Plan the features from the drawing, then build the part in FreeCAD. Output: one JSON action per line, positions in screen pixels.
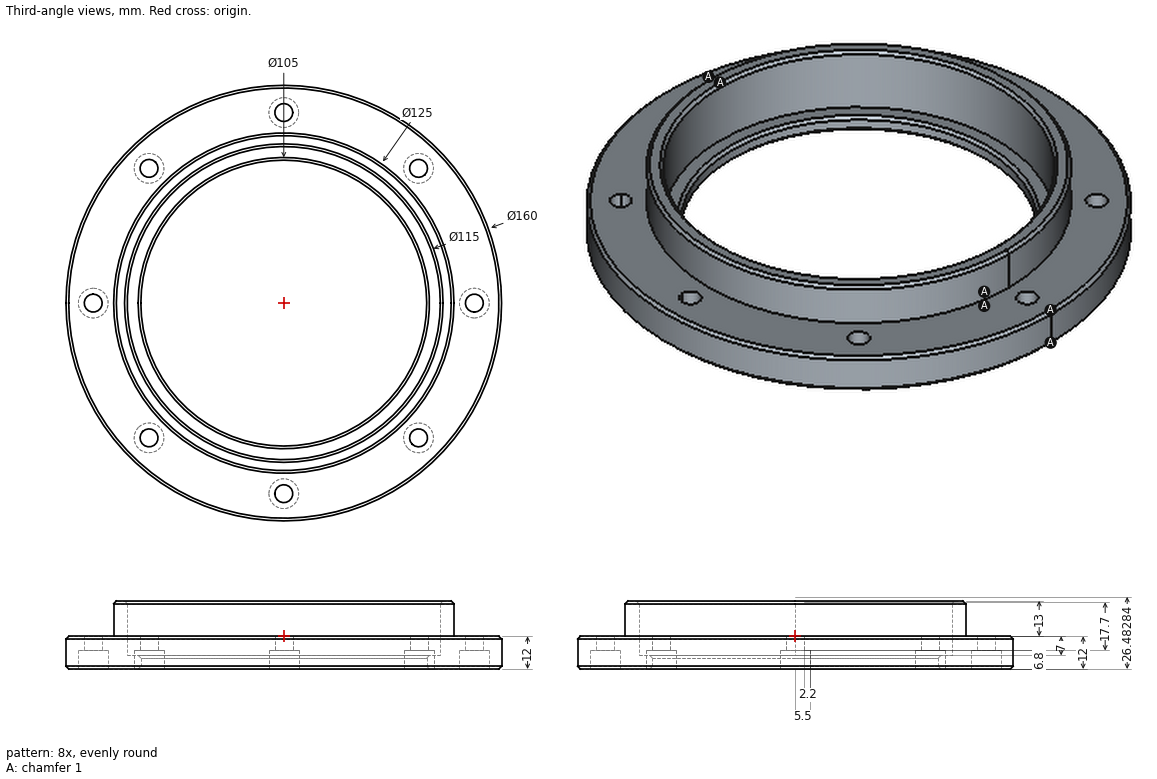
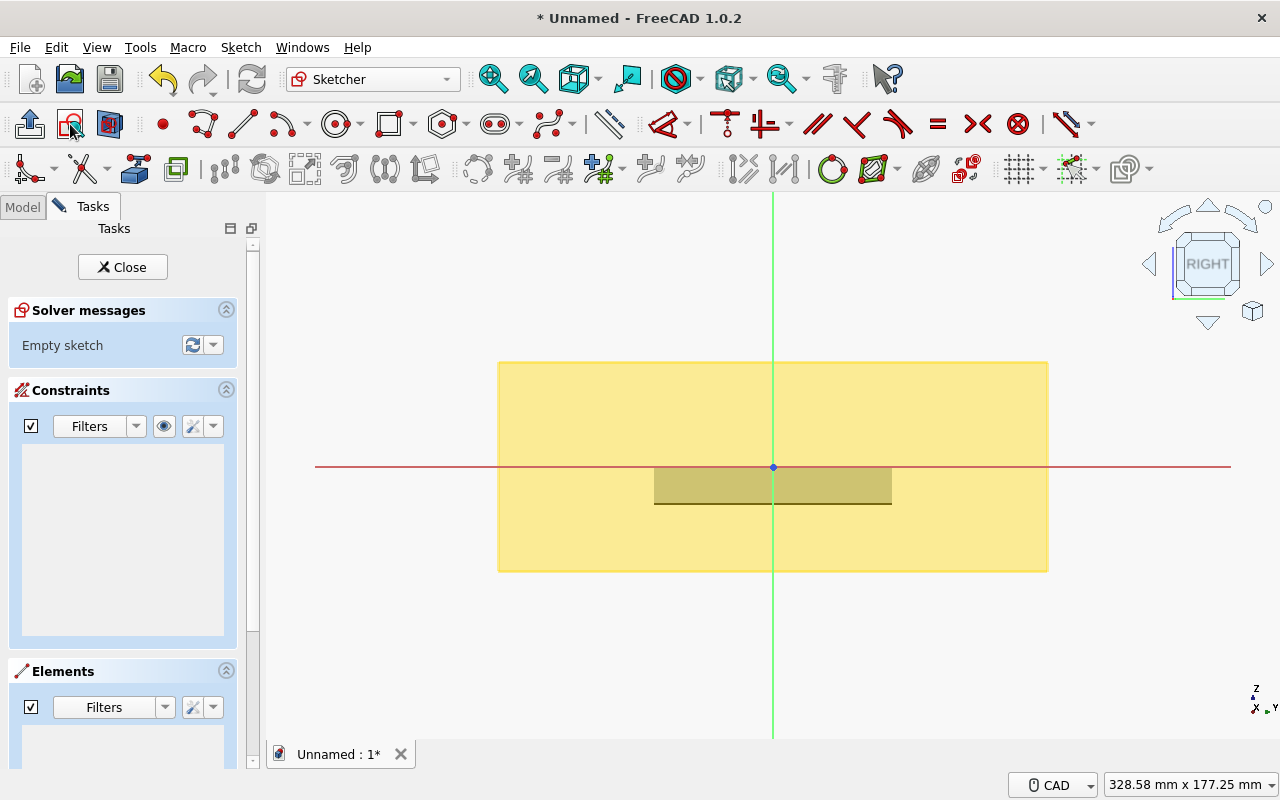
{"action": "scroll", "coordinate": [807, 462], "scroll_direction": "up", "scroll_amount": 7}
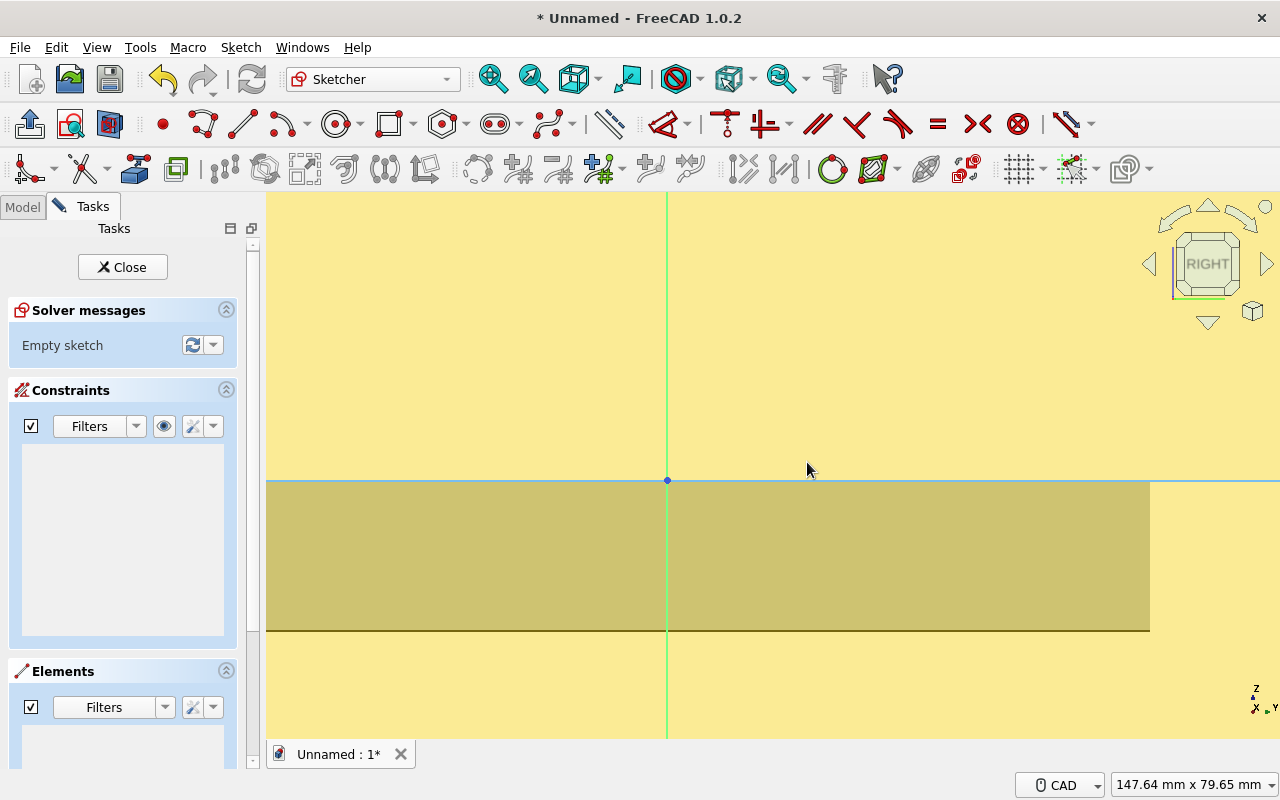
{"action": "key", "text": "g m"}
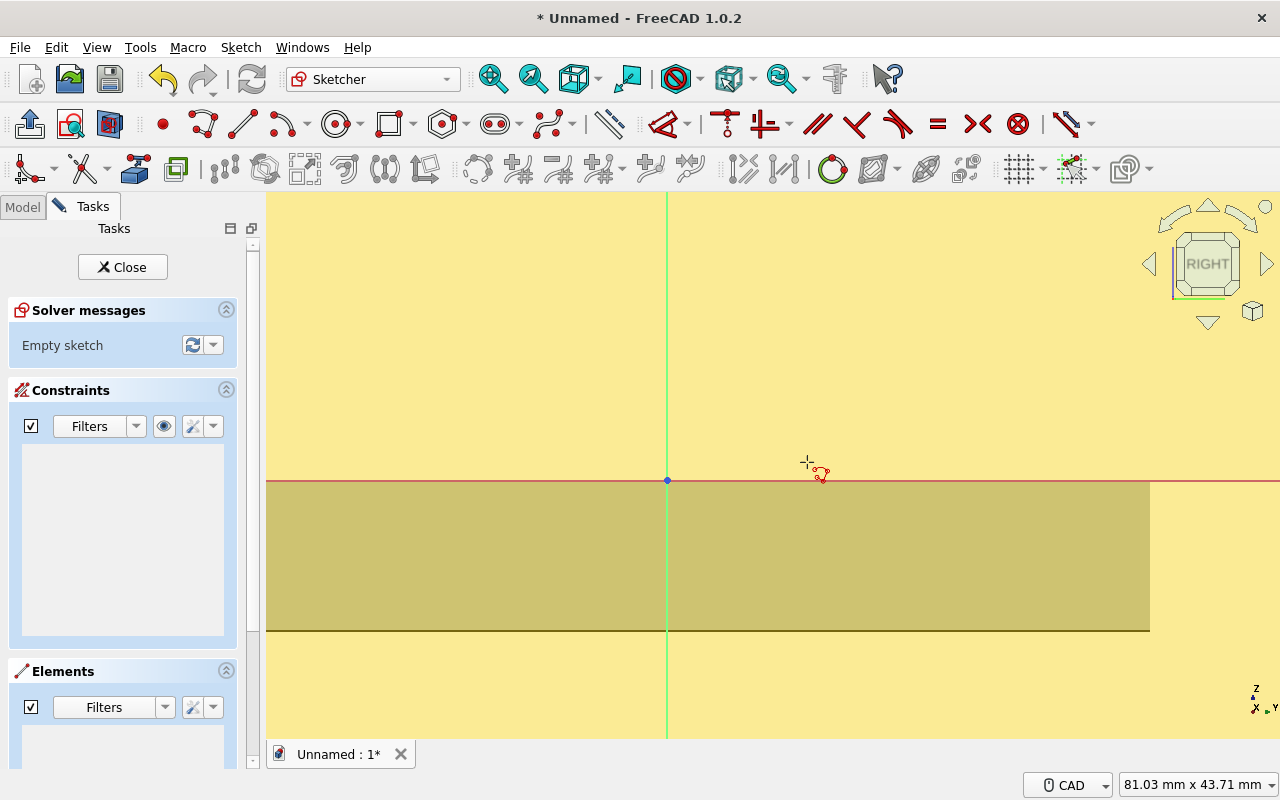
{"action": "left_click", "coordinate": [709, 546]}
{"action": "left_click", "coordinate": [709, 325]}
{"action": "left_click", "coordinate": [667, 300]}
{"action": "left_click", "coordinate": [676, 631]}
{"action": "left_click", "coordinate": [736, 631]}
{"action": "left_click", "coordinate": [736, 546]}
{"action": "left_click", "coordinate": [709, 547]}
{"action": "key", "text": "Escape"}
{"action": "key", "text": "Escape"}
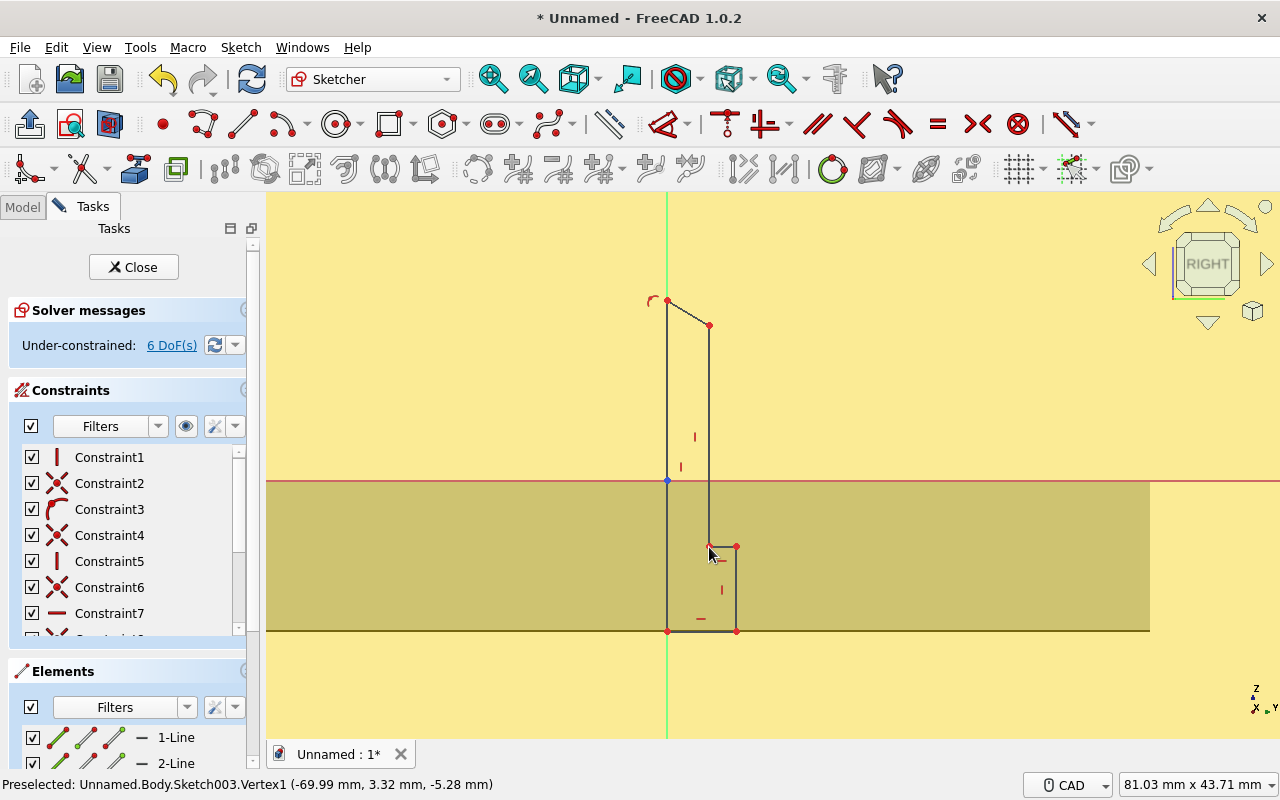
{"action": "left_click", "coordinate": [688, 632]}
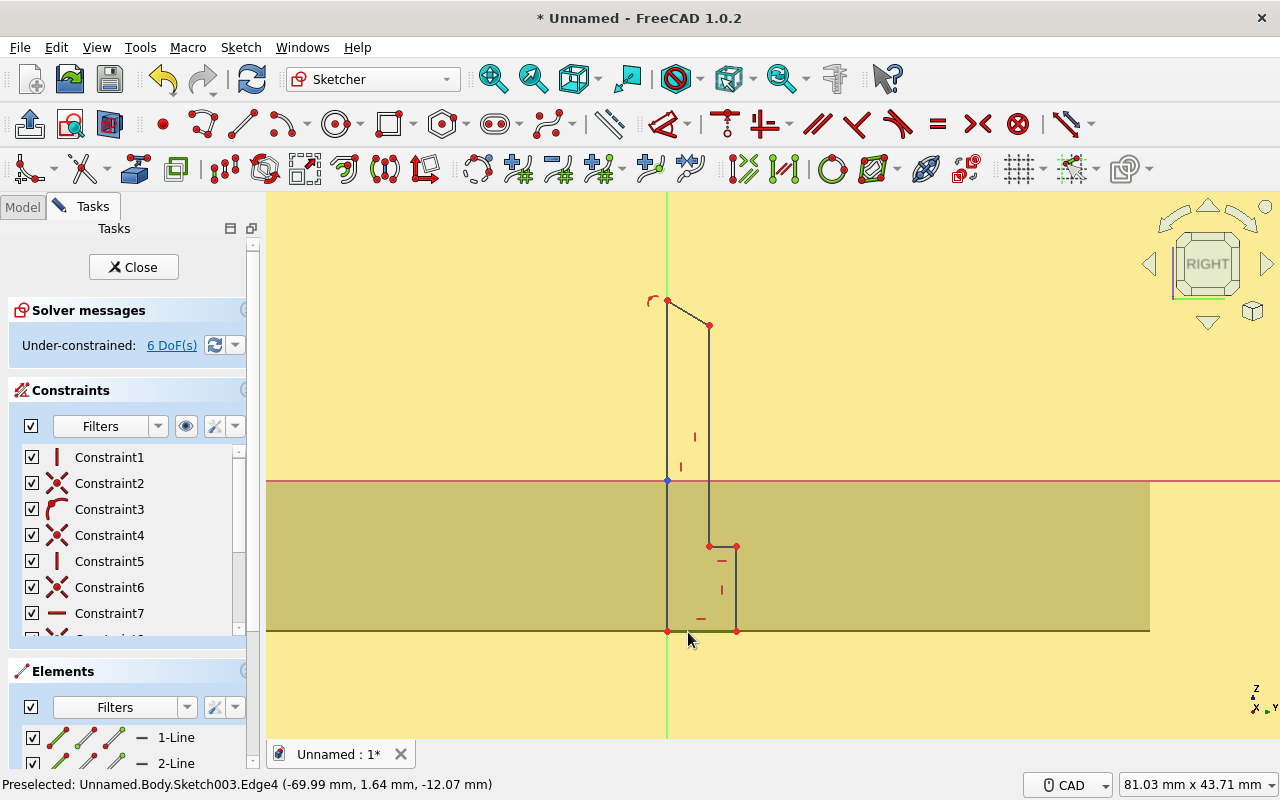
{"action": "key", "text": "l"}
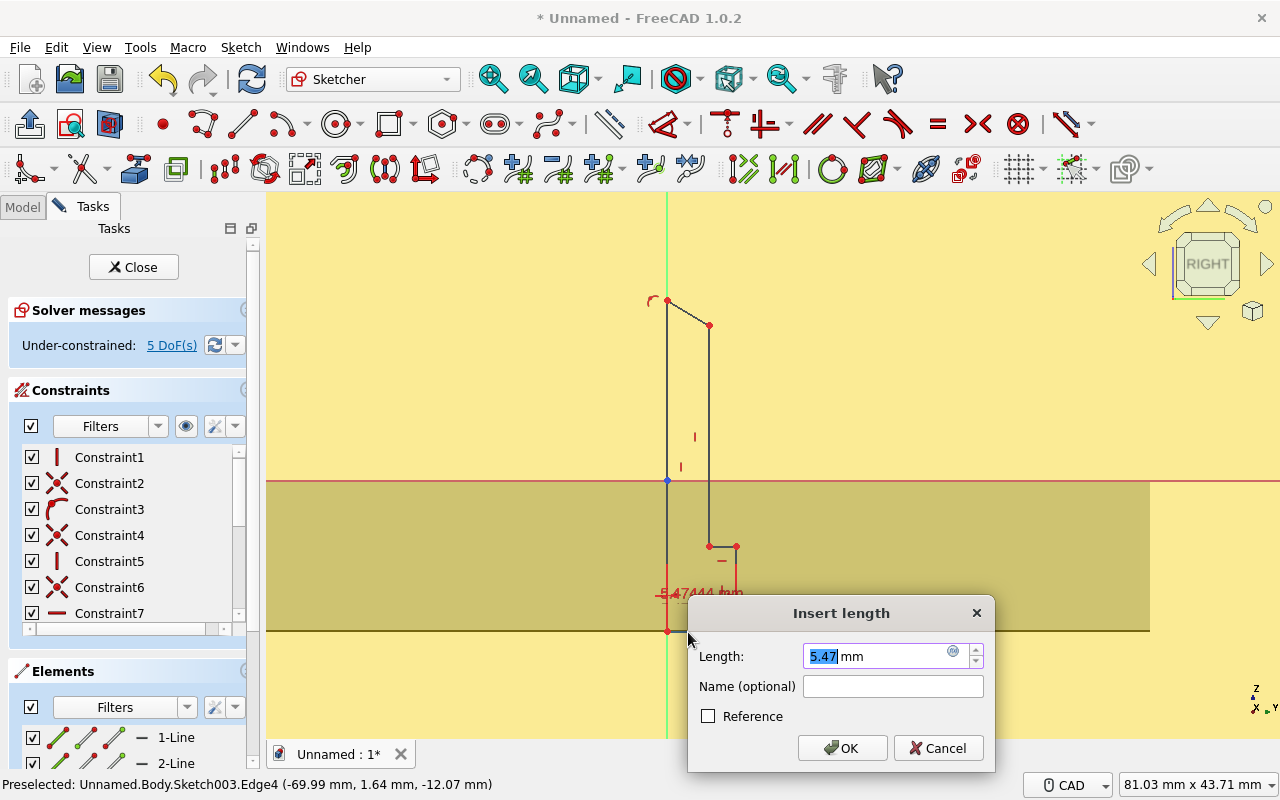
{"action": "type", "text": "5.5"}
{"action": "key", "text": "Return"}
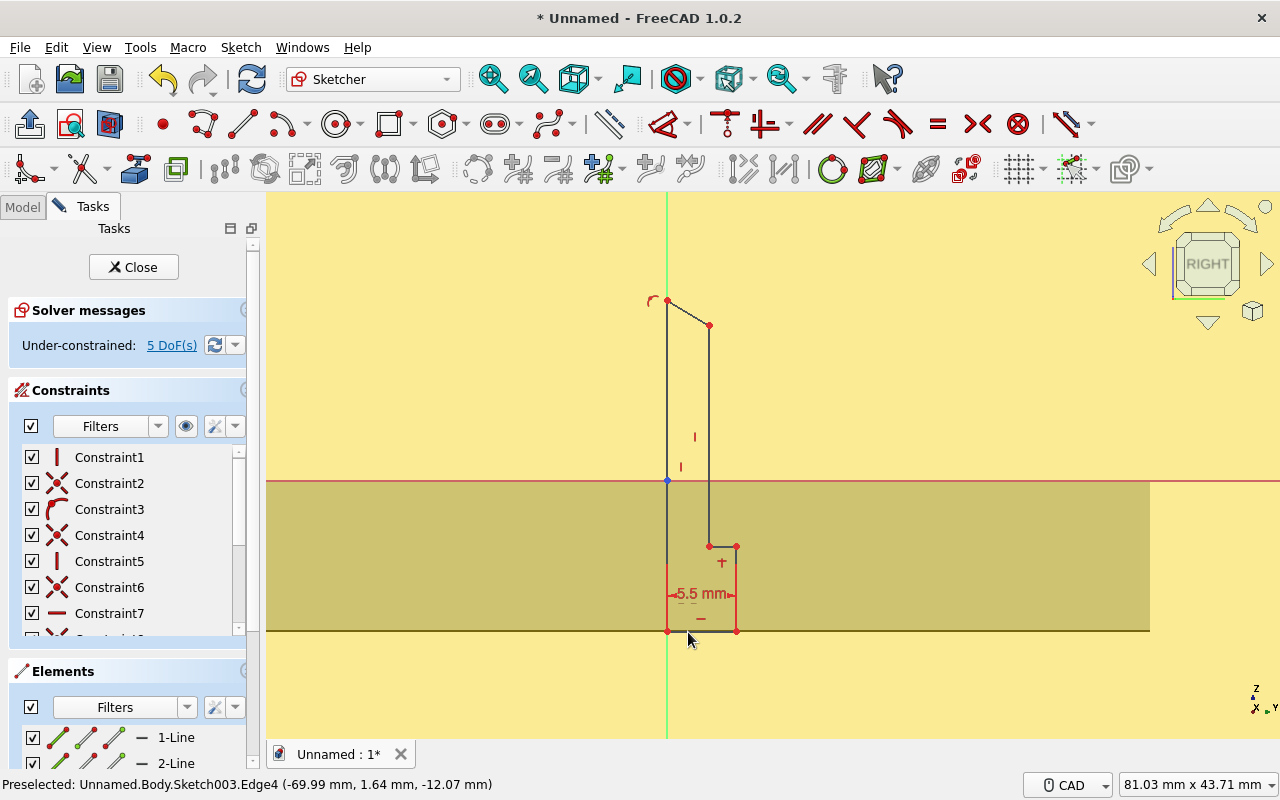
{"action": "left_click", "coordinate": [736, 607]}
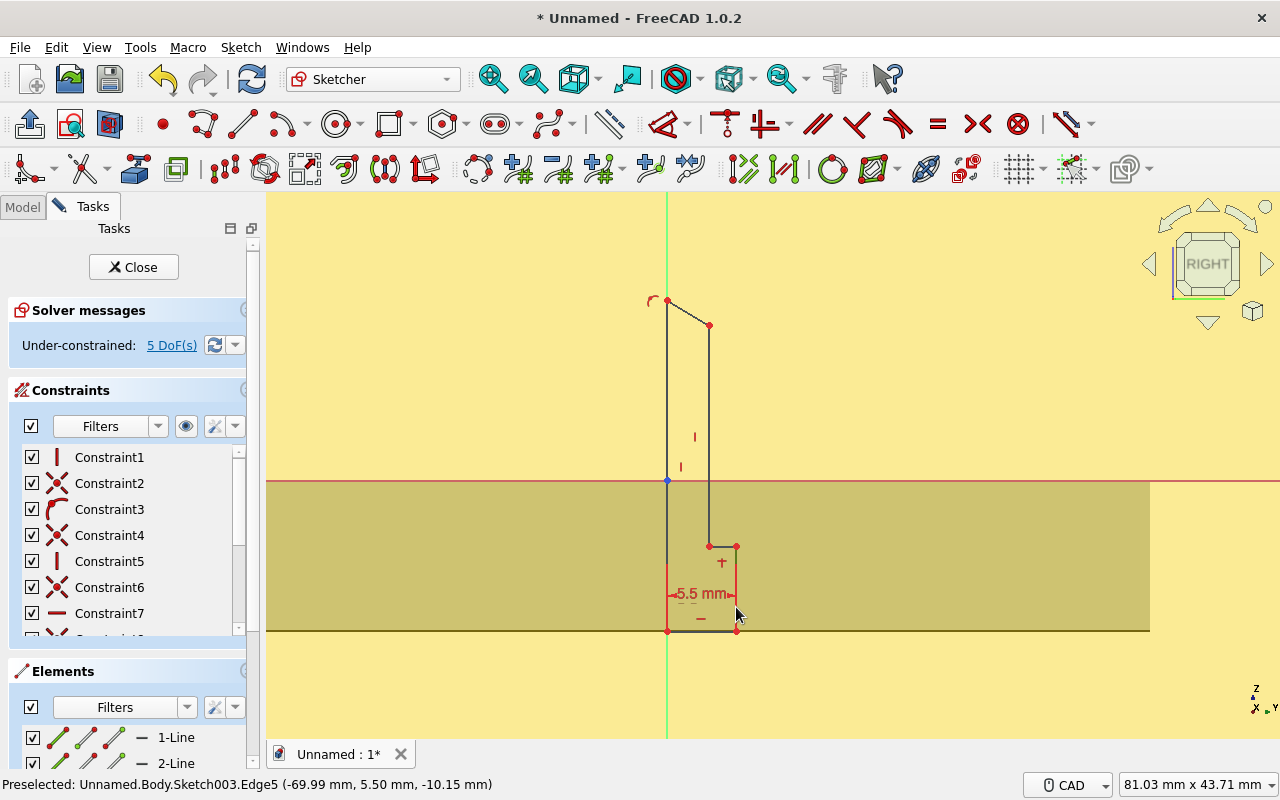
{"action": "key", "text": "i"}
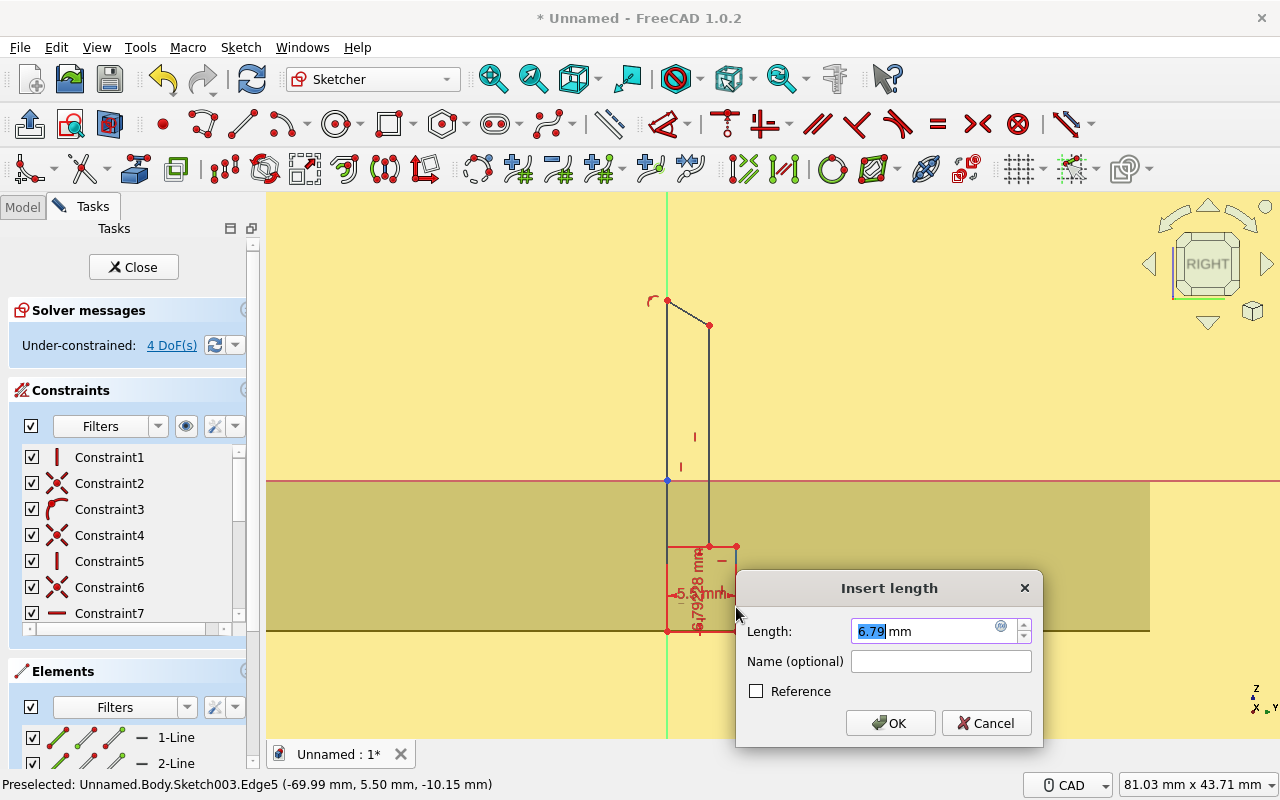
{"action": "type", "text": "6.8"}
{"action": "key", "text": "Return"}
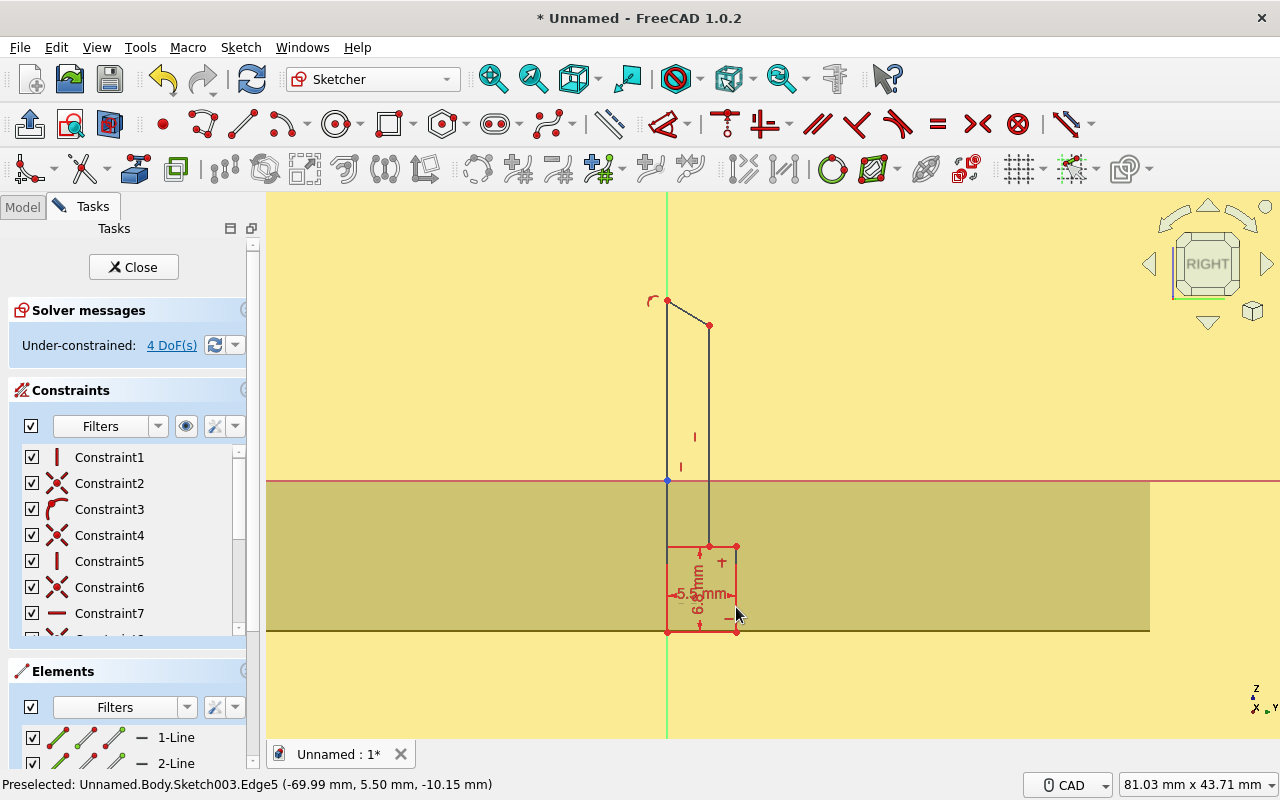
{"action": "scroll", "coordinate": [725, 547], "scroll_direction": "up", "scroll_amount": 2}